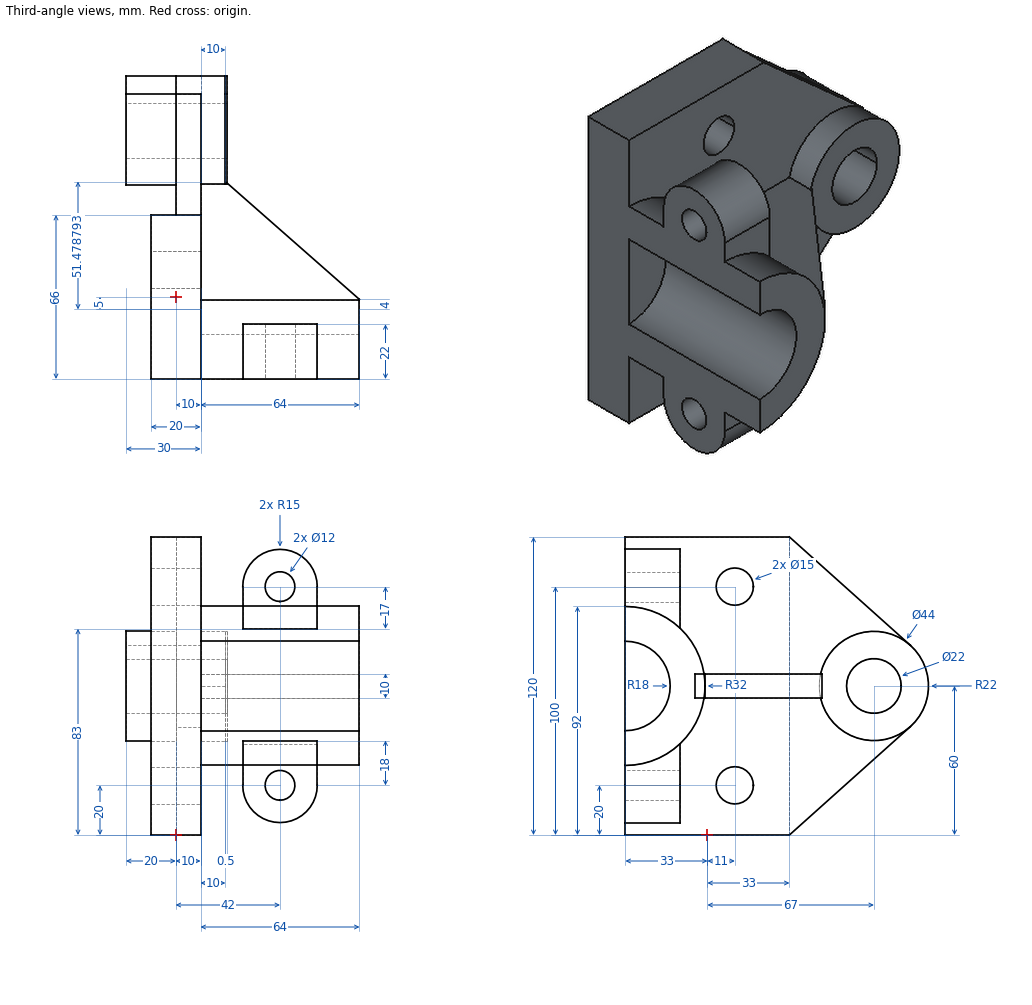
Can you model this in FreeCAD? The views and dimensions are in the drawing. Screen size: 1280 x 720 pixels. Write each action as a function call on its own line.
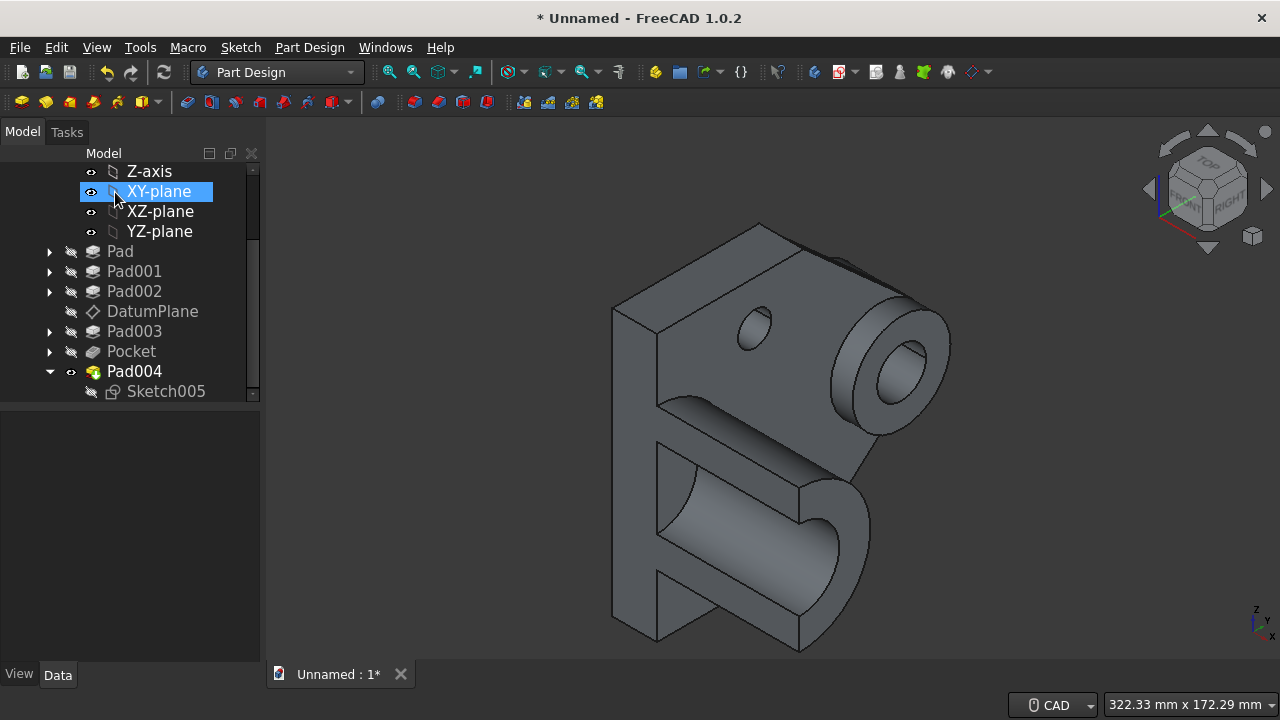
click(390, 72)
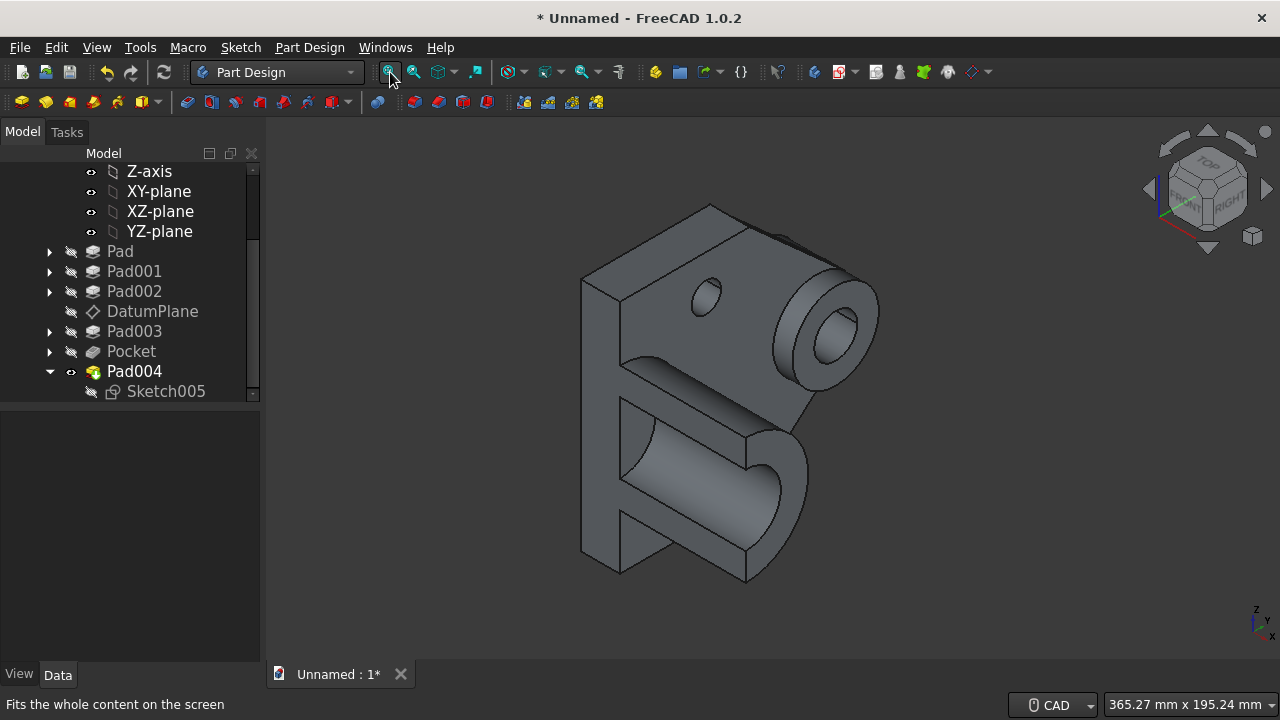
click(816, 72)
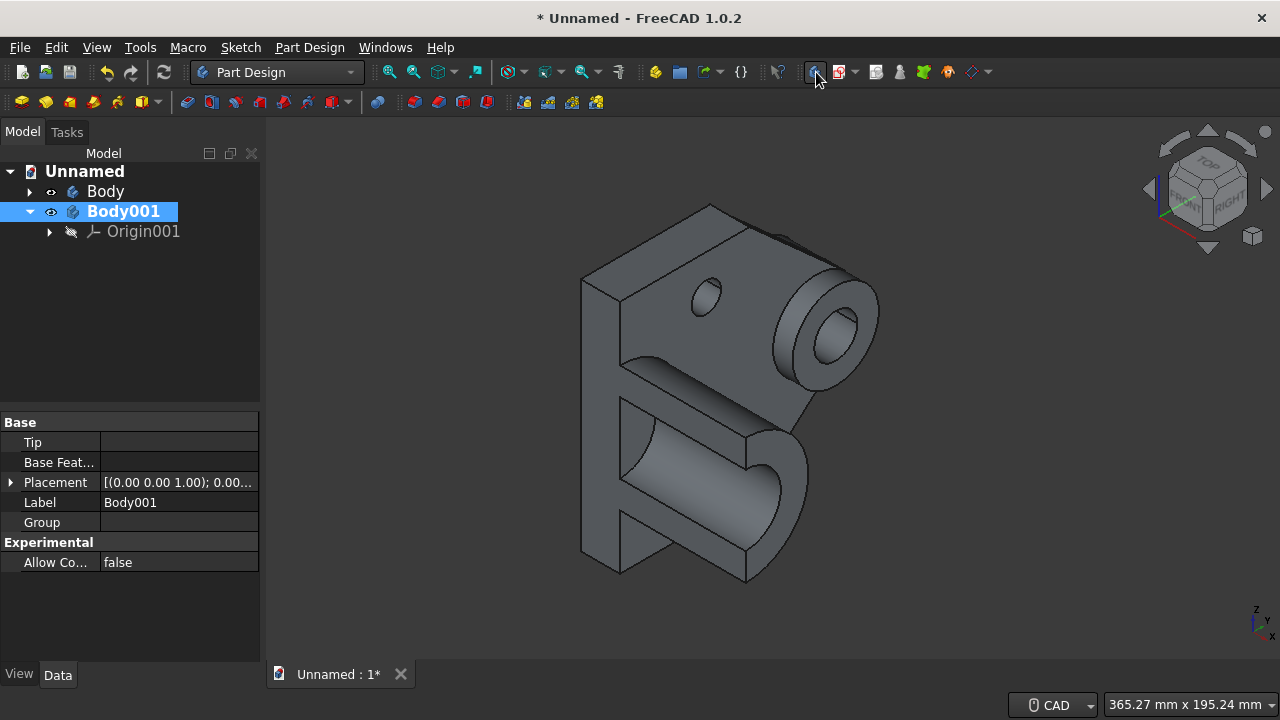
click(50, 232)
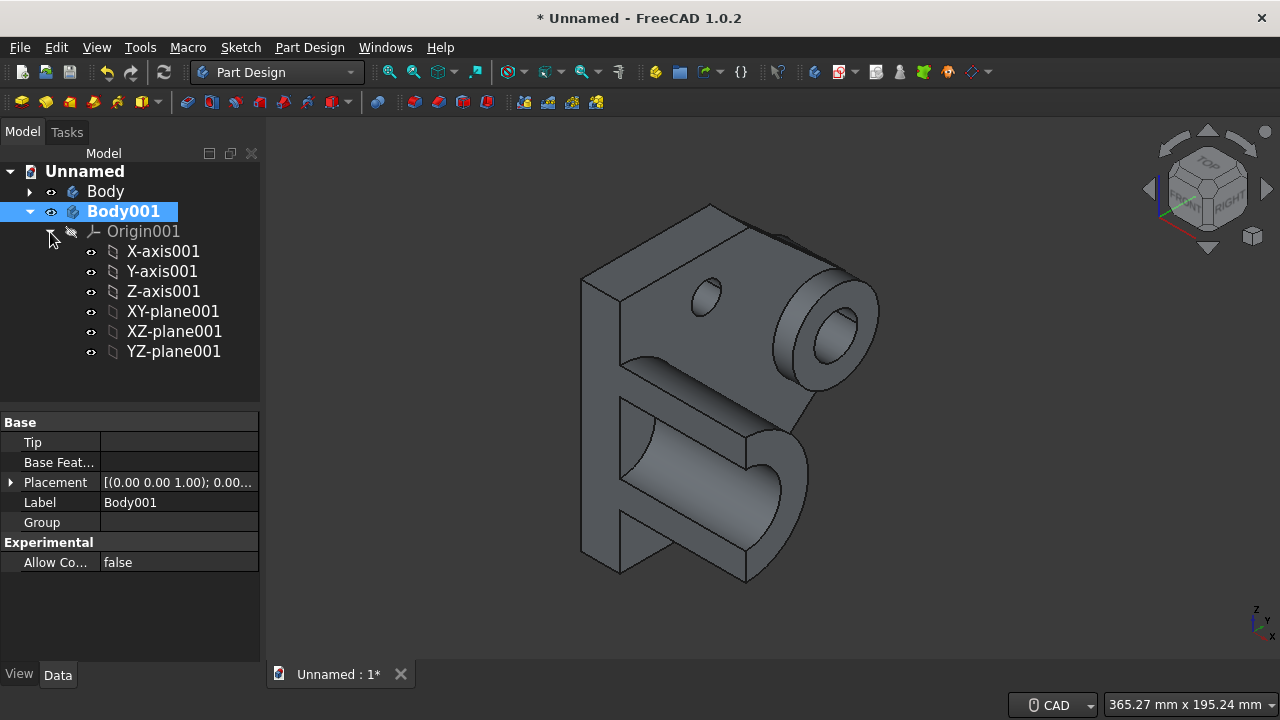
click(136, 312)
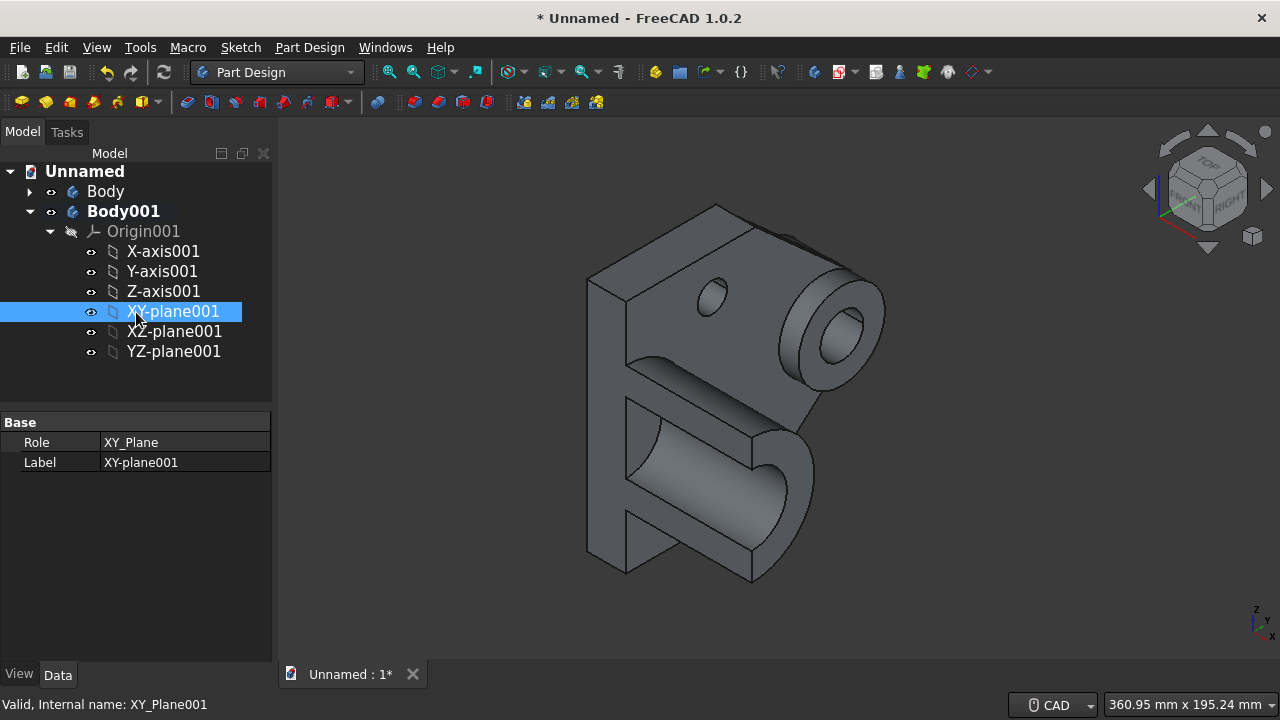
click(972, 72)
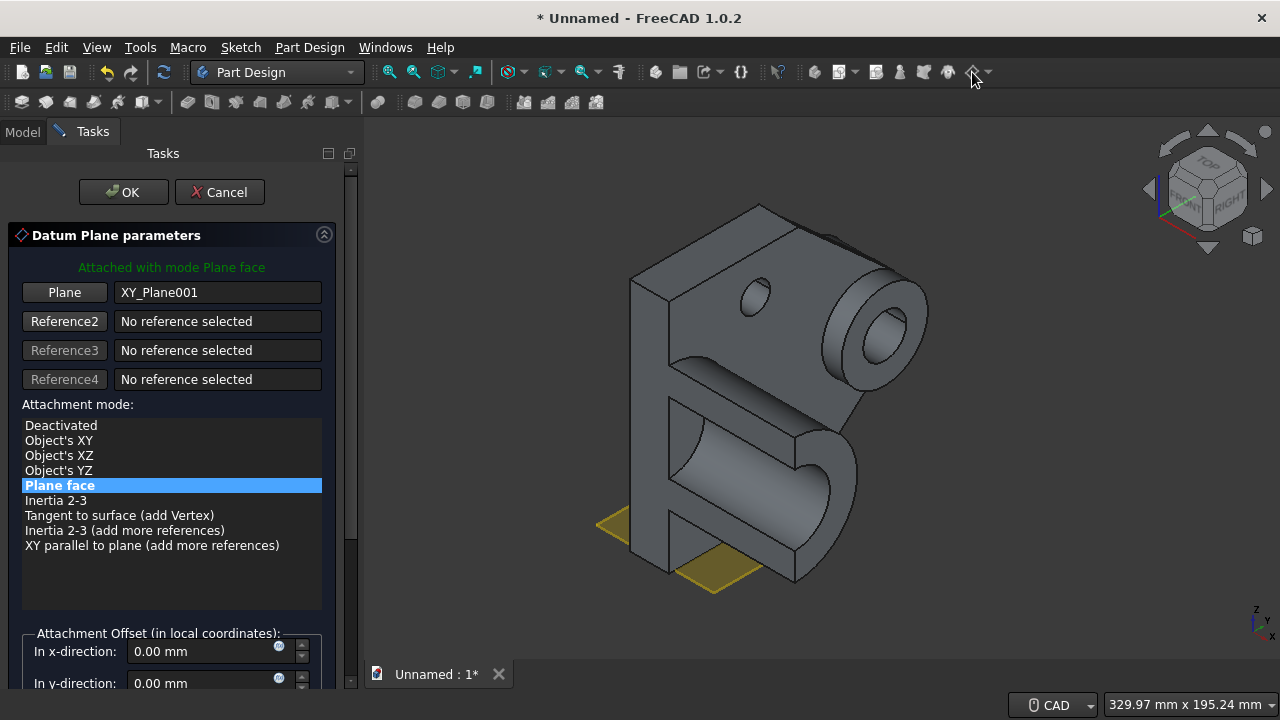
scroll(351, 426, down, 2)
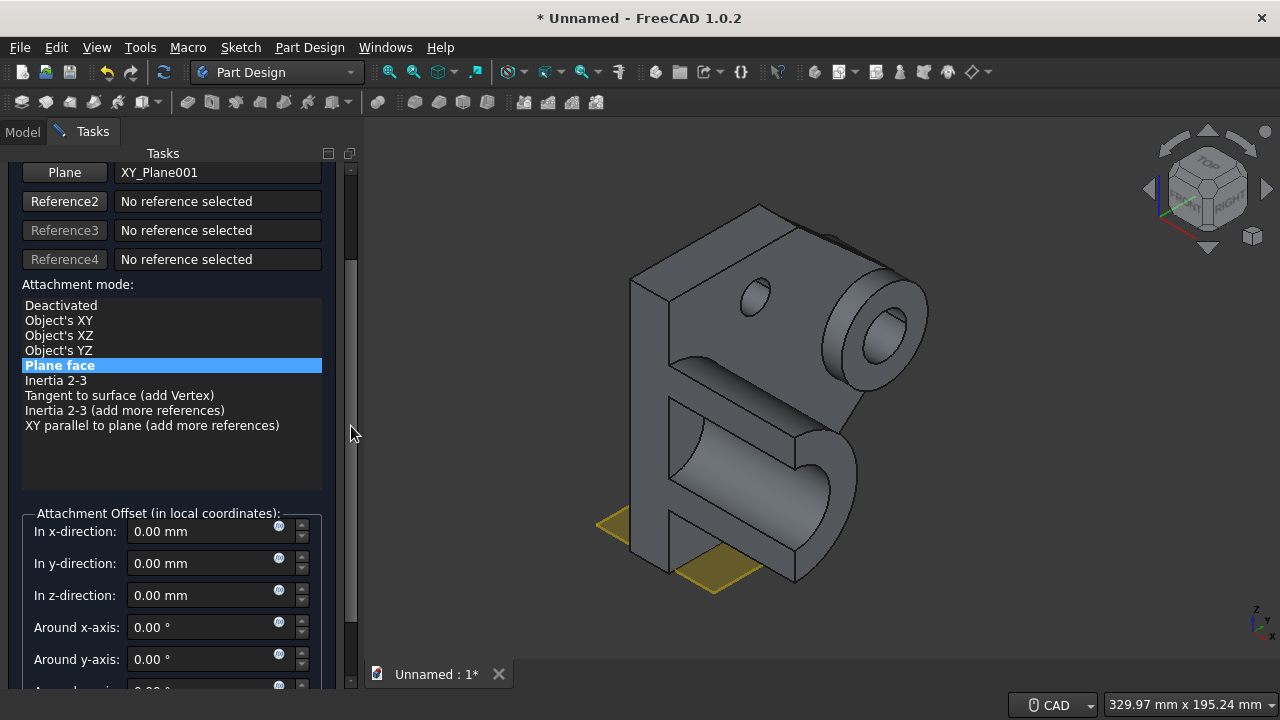
triple_click(210, 595)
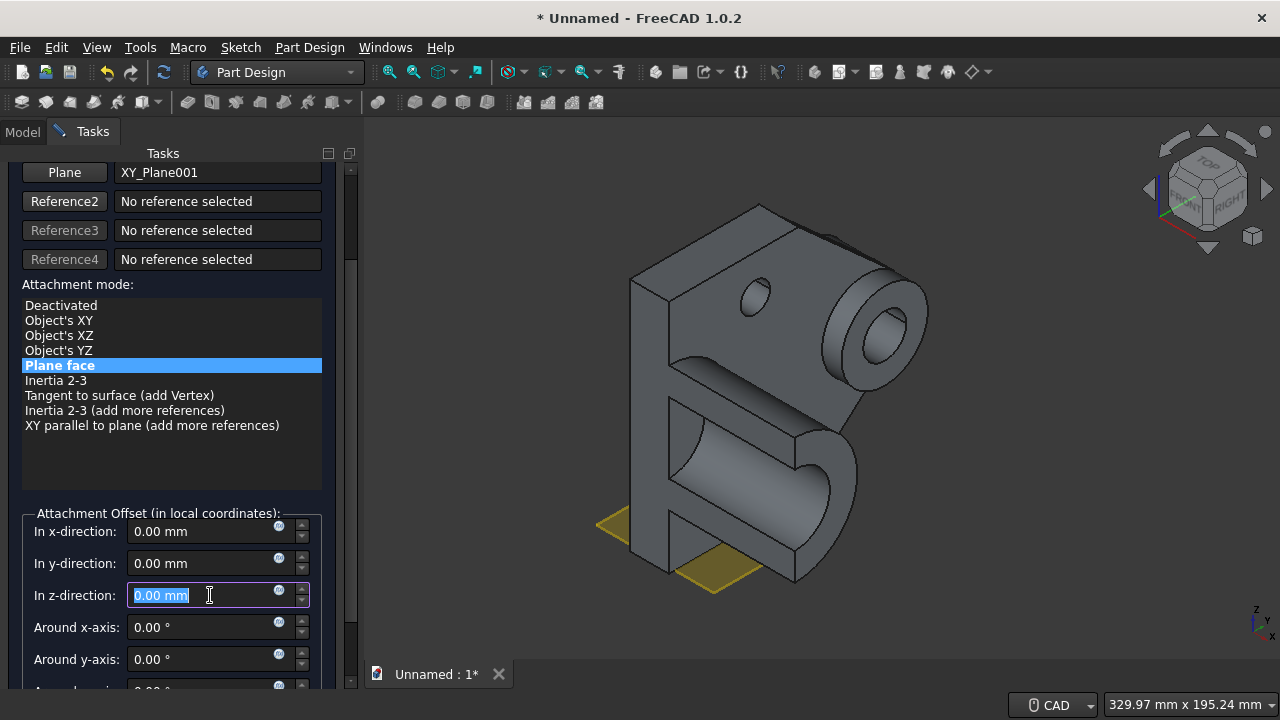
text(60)
key(Tab)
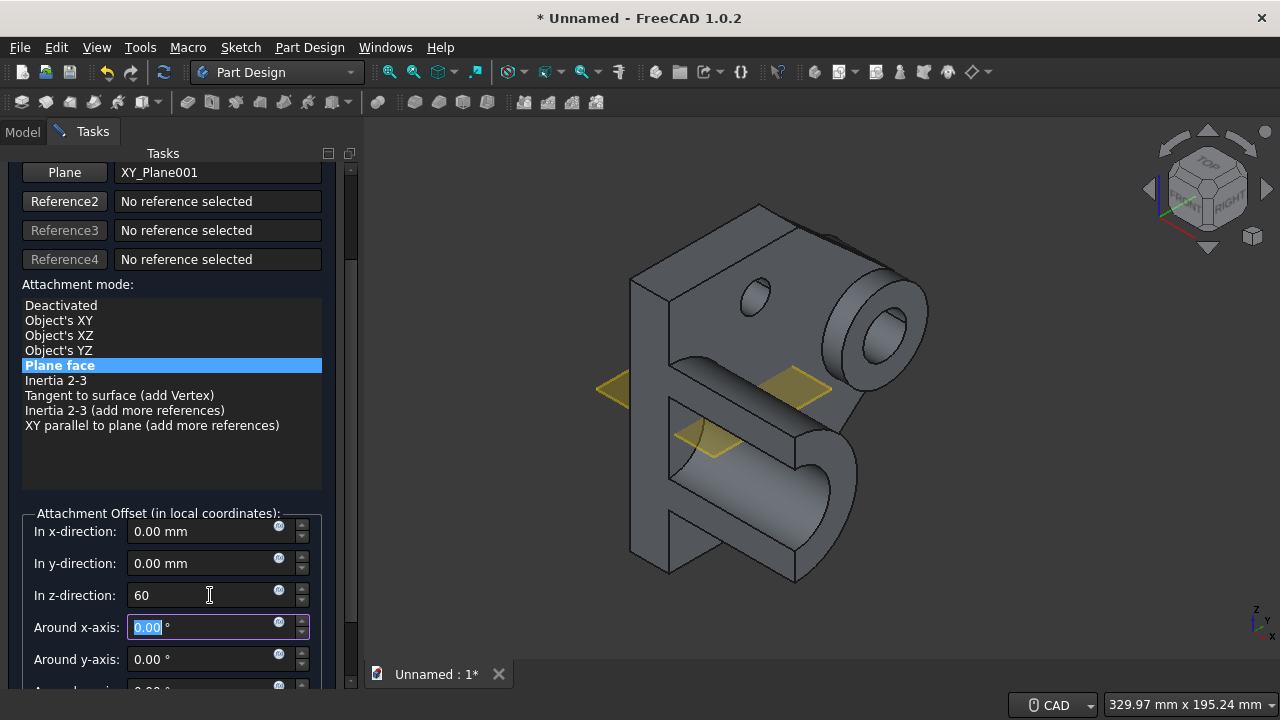
scroll(351, 426, up, 3)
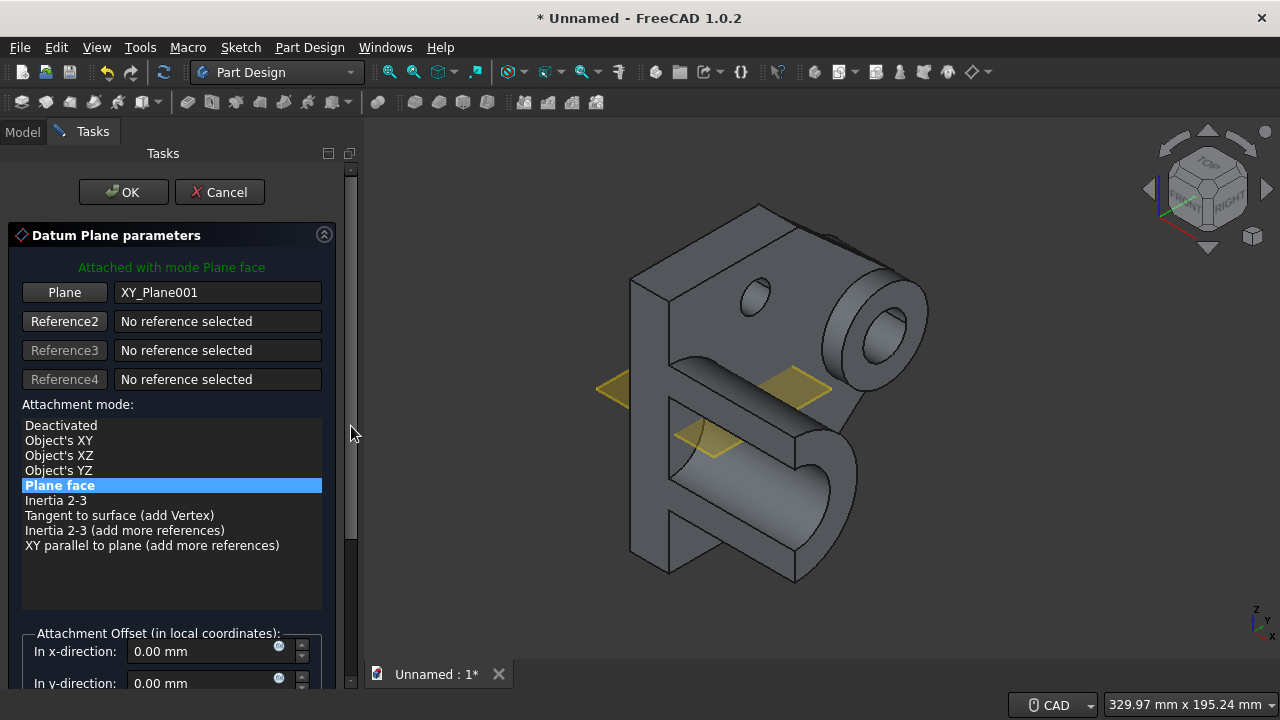
click(124, 192)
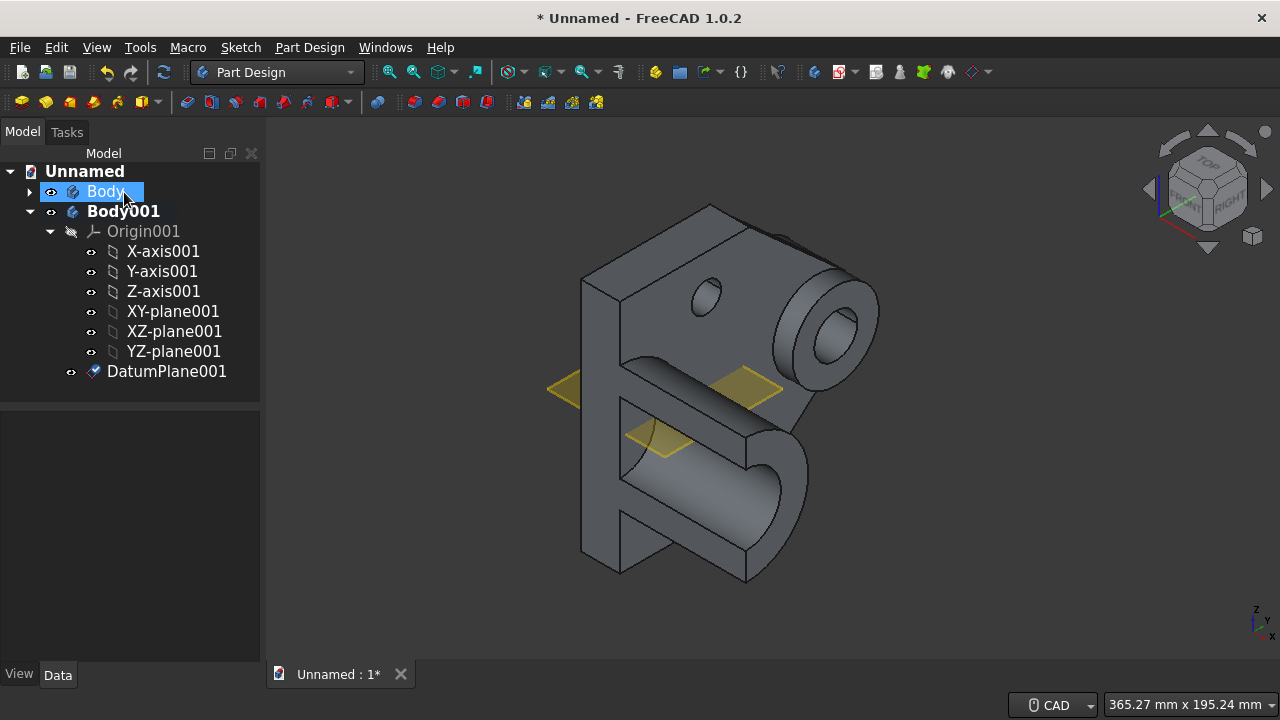
click(116, 372)